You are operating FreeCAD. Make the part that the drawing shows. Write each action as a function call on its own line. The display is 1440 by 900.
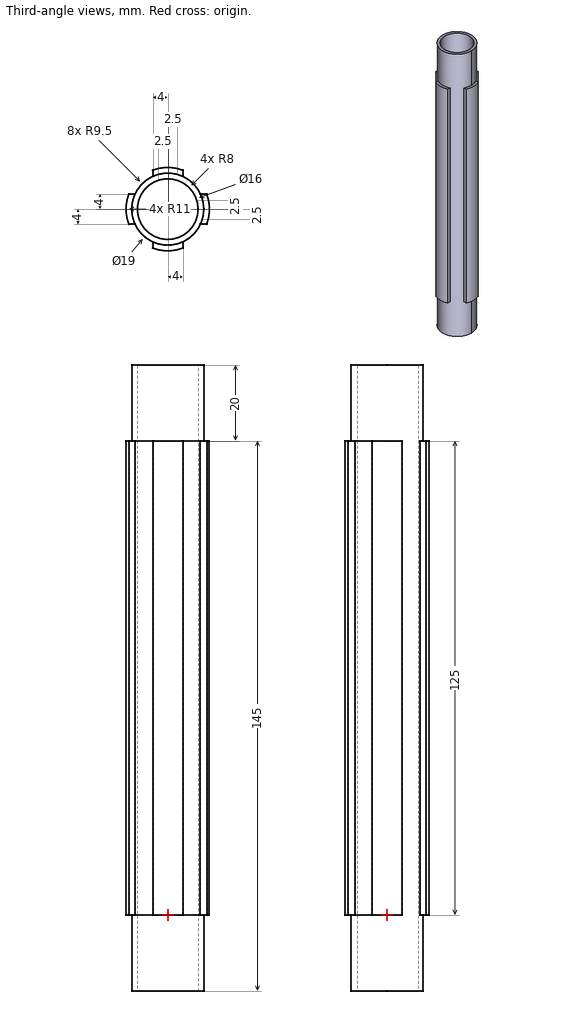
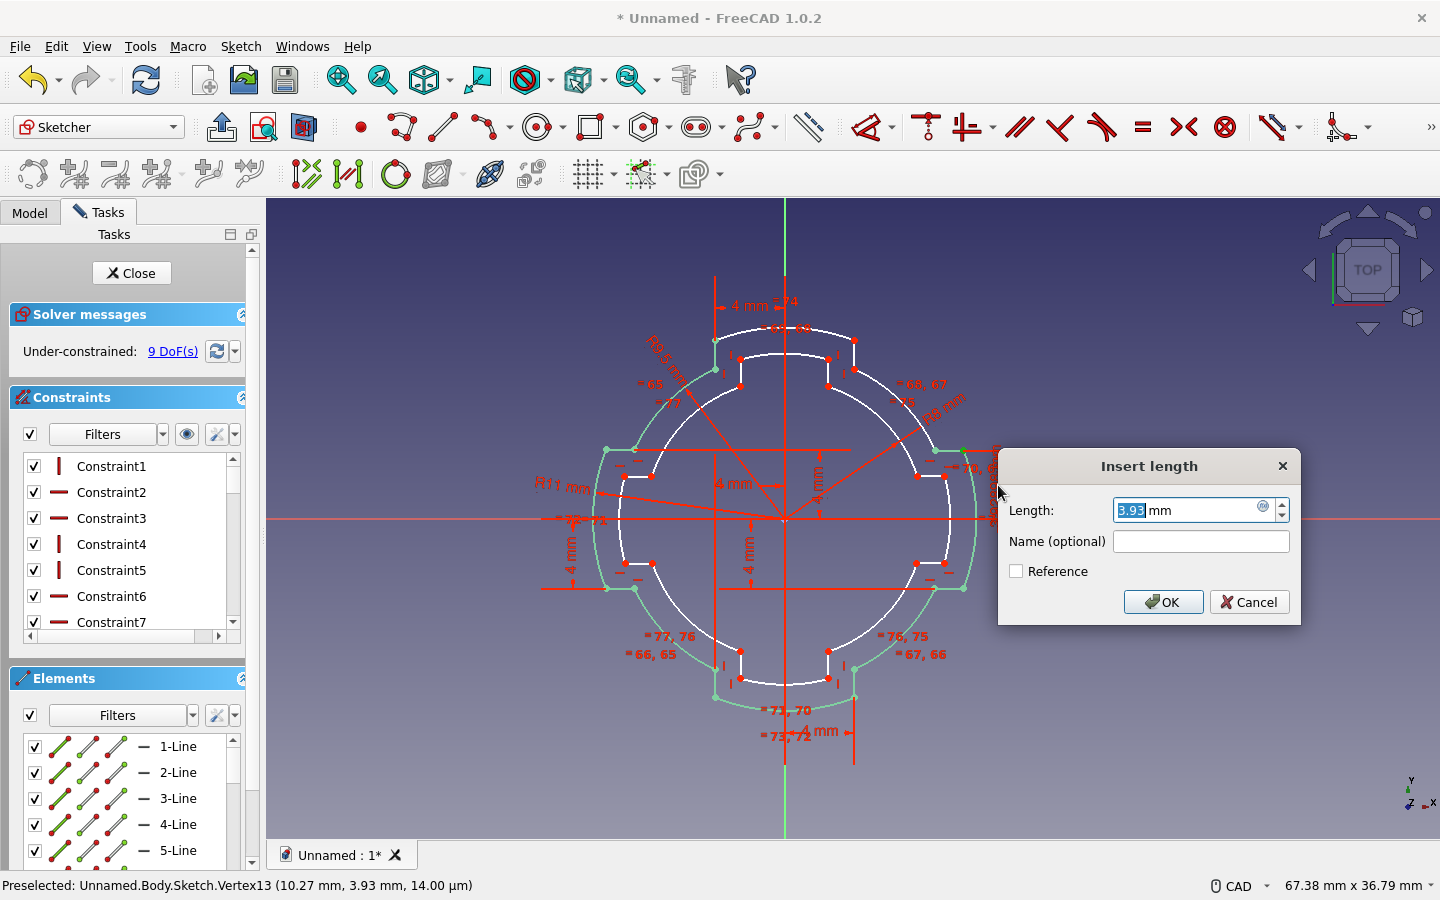
text(4)
key(Return)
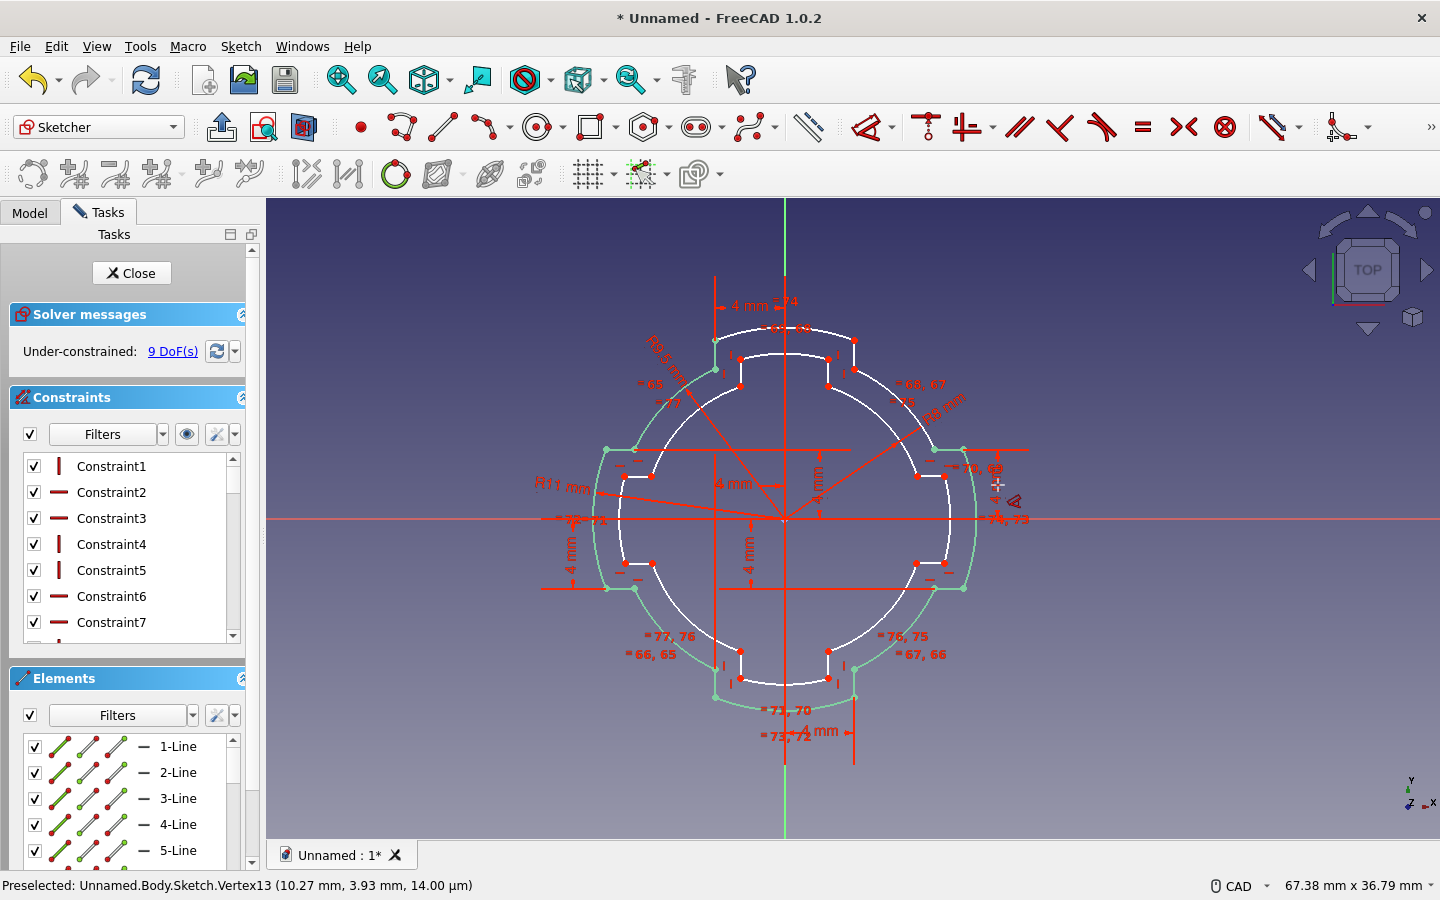
click(854, 369)
click(836, 553)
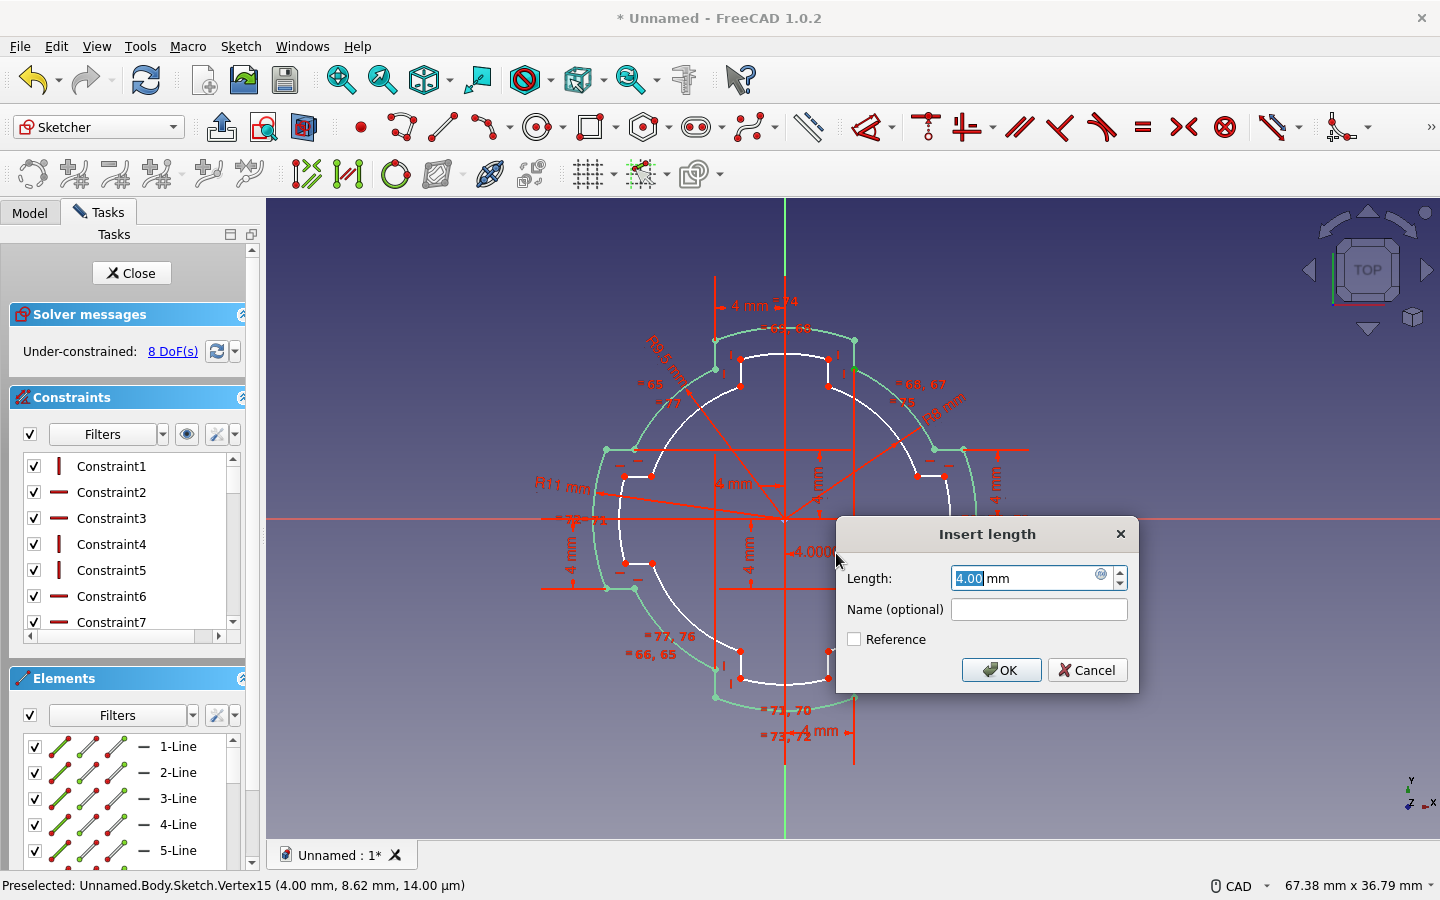
text(4)
key(Return)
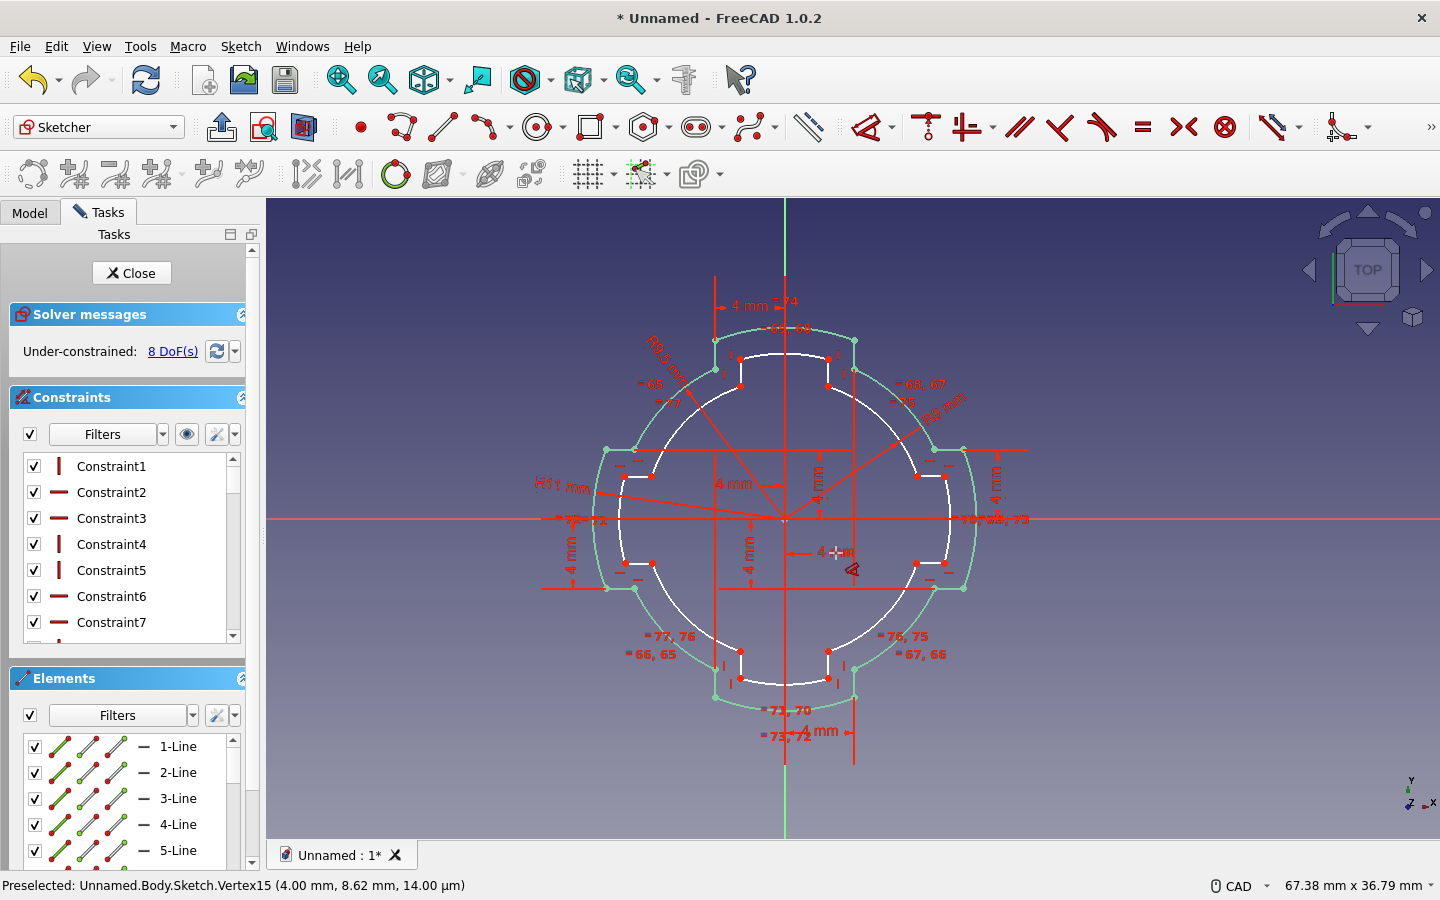
click(741, 387)
click(763, 577)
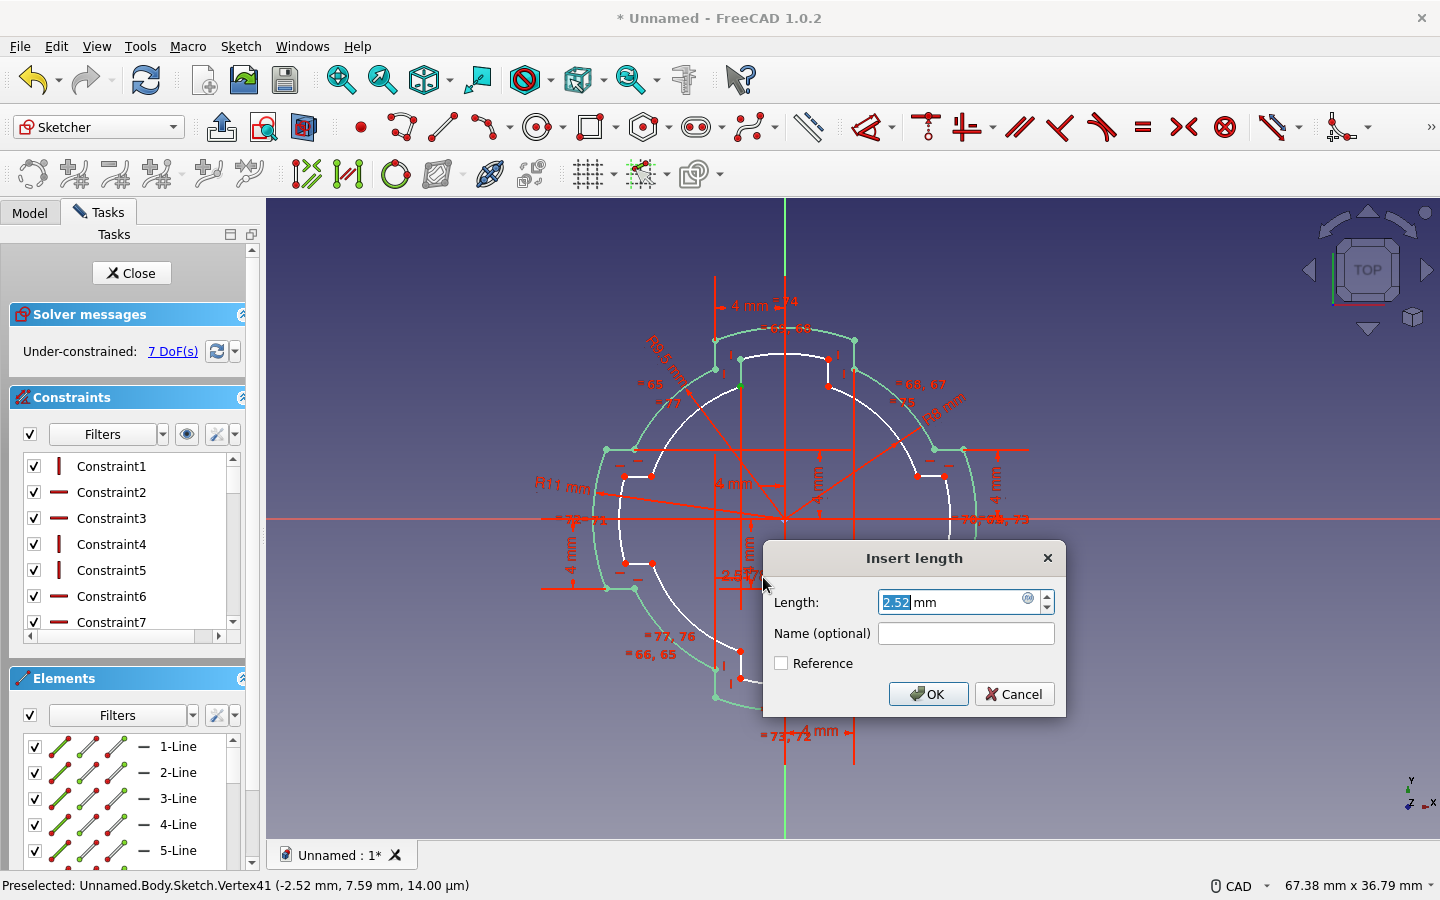
text(2.5)
key(Return)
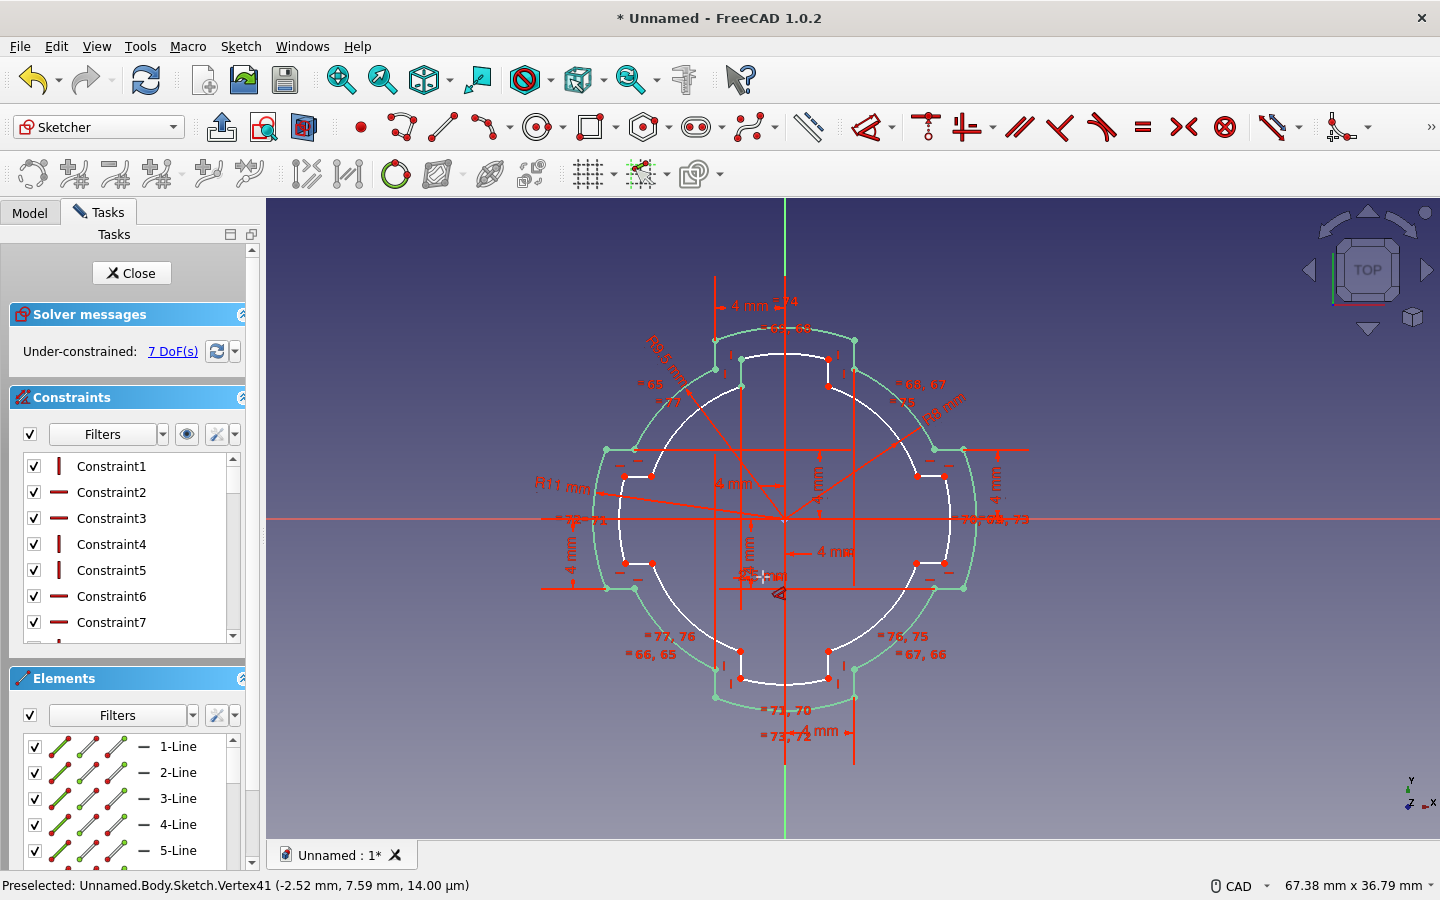
click(828, 359)
click(822, 301)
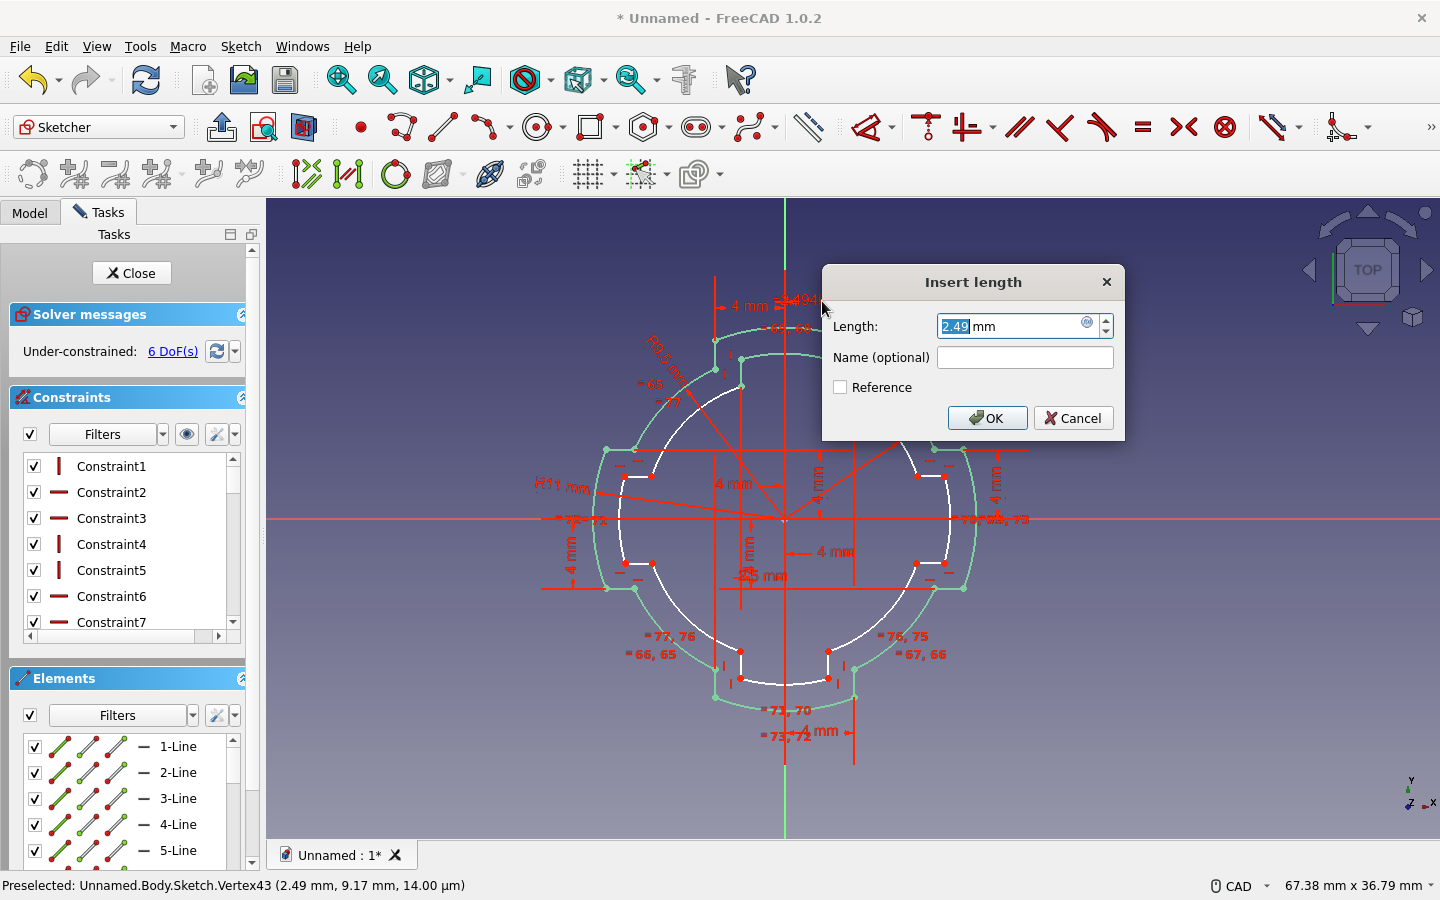
text(2.5)
key(Return)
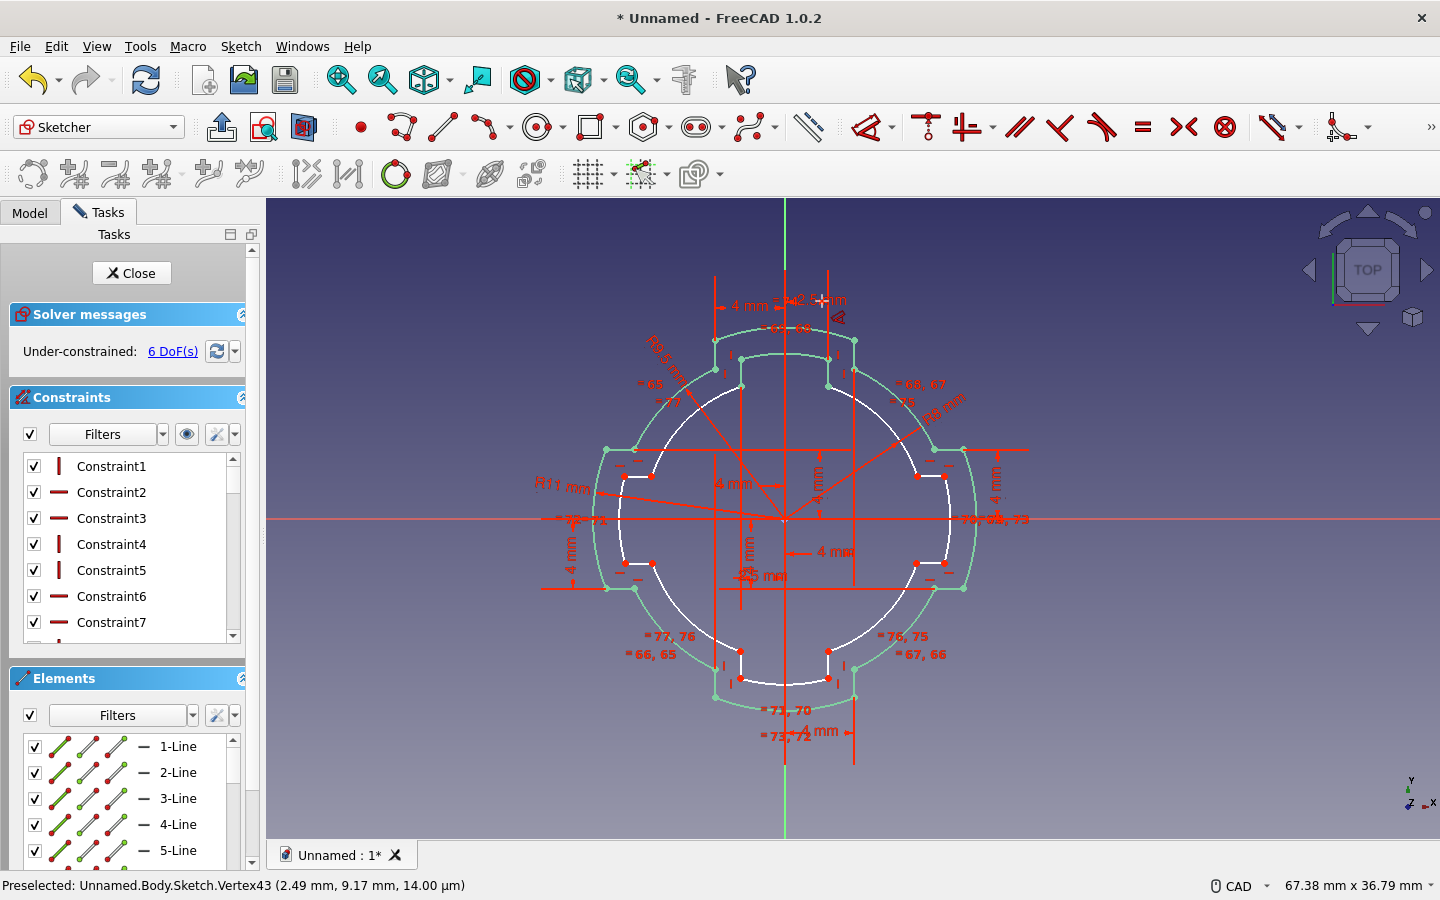
click(917, 476)
click(655, 498)